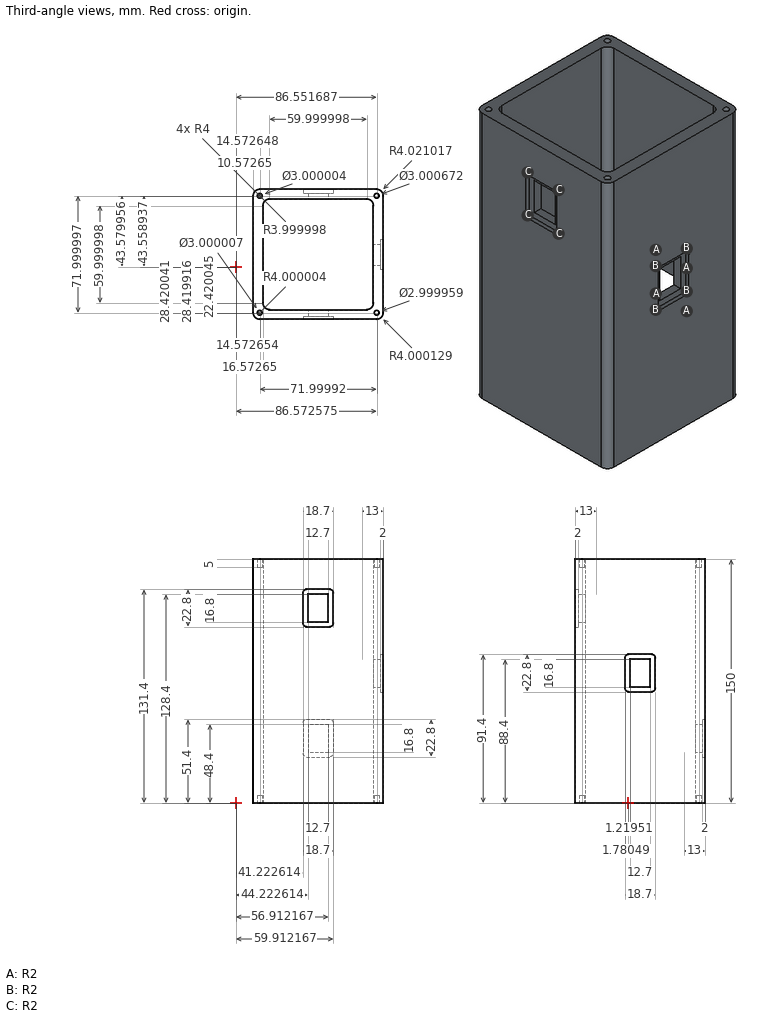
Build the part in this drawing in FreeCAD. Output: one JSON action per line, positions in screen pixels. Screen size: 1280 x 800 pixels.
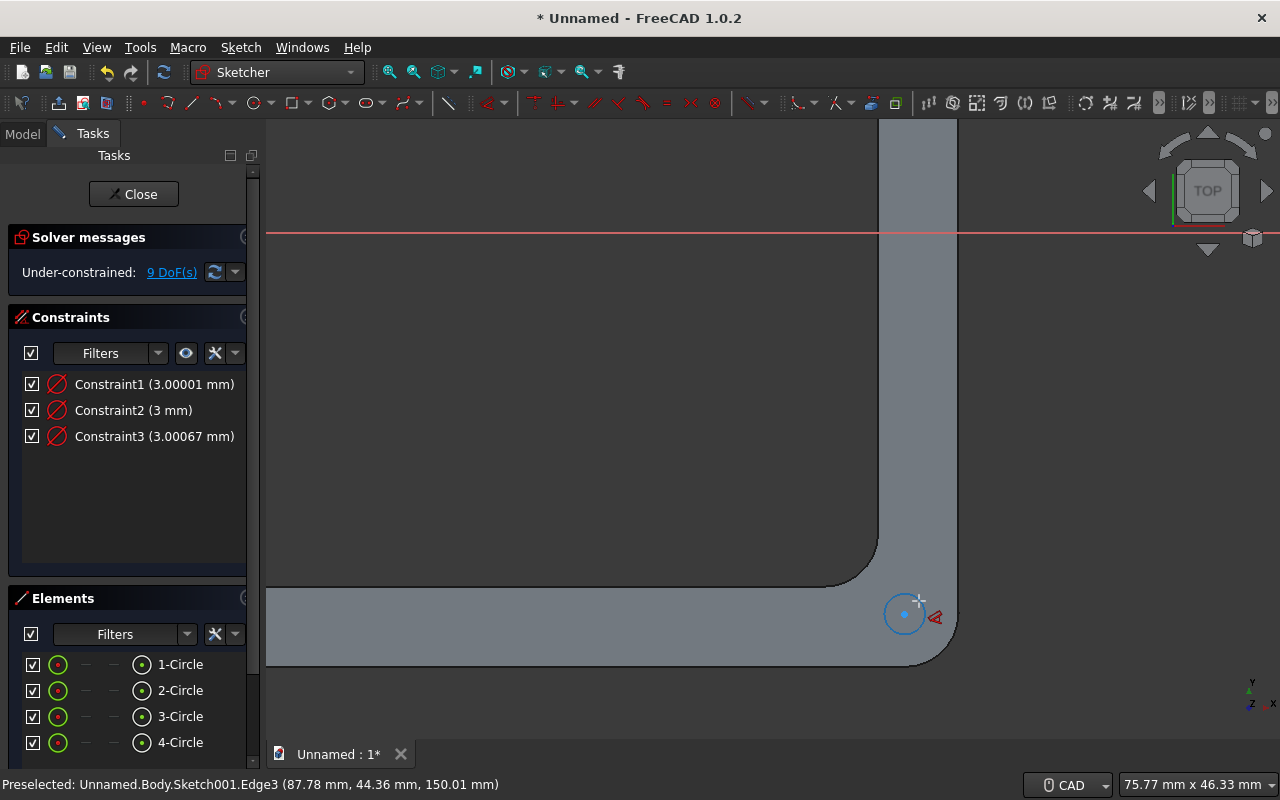
{"action": "left_click", "coordinate": [919, 600]}
{"action": "left_click", "coordinate": [942, 578]}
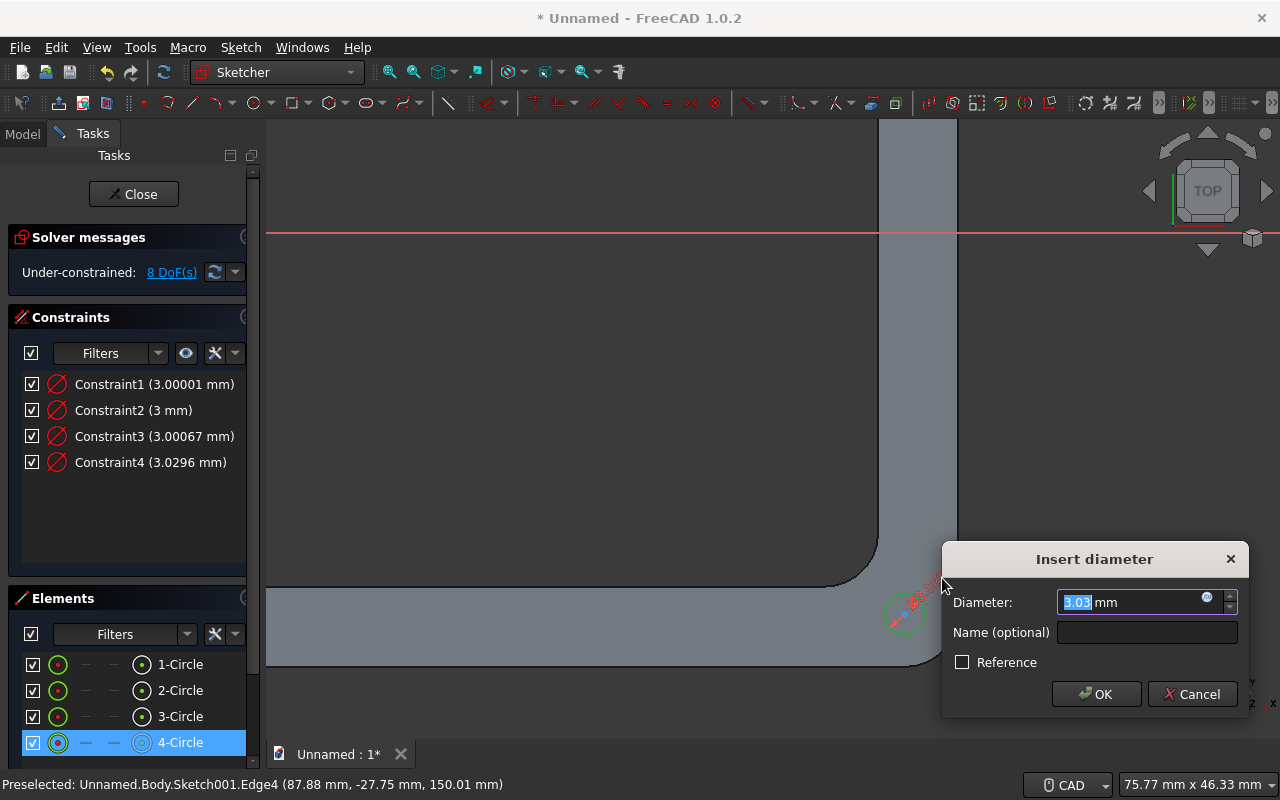
{"action": "type", "text": "2.999959"}
{"action": "key", "text": "Return"}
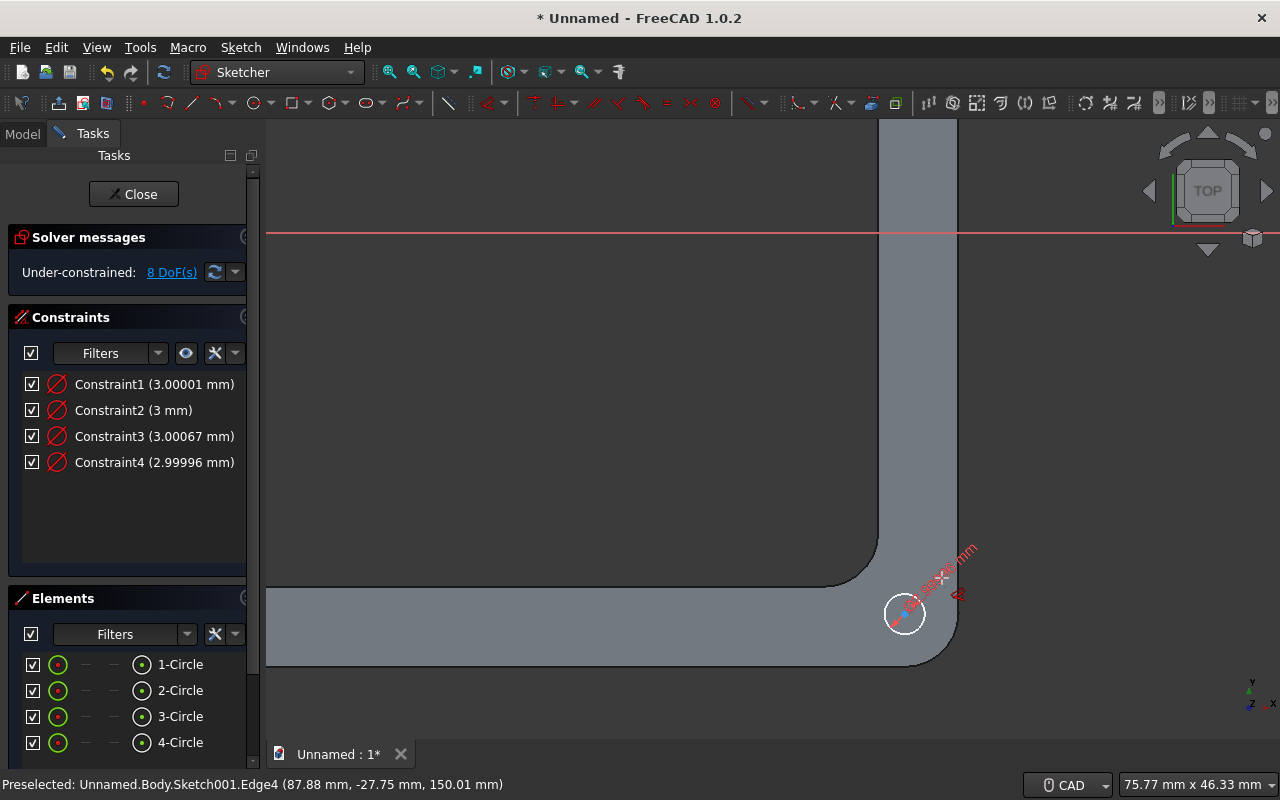
{"action": "scroll", "coordinate": [919, 602], "scroll_direction": "down", "scroll_amount": 5}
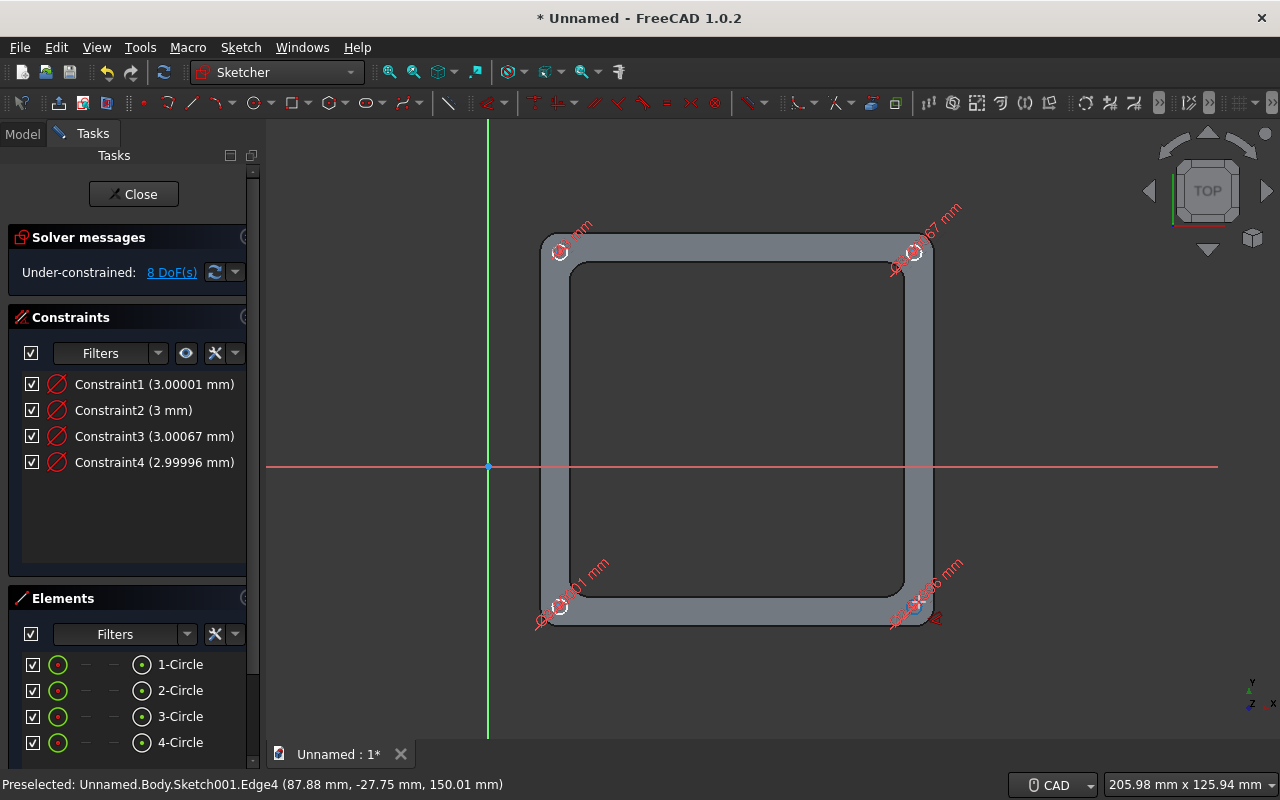
{"action": "left_click", "coordinate": [560, 607]}
{"action": "left_click", "coordinate": [524, 641]}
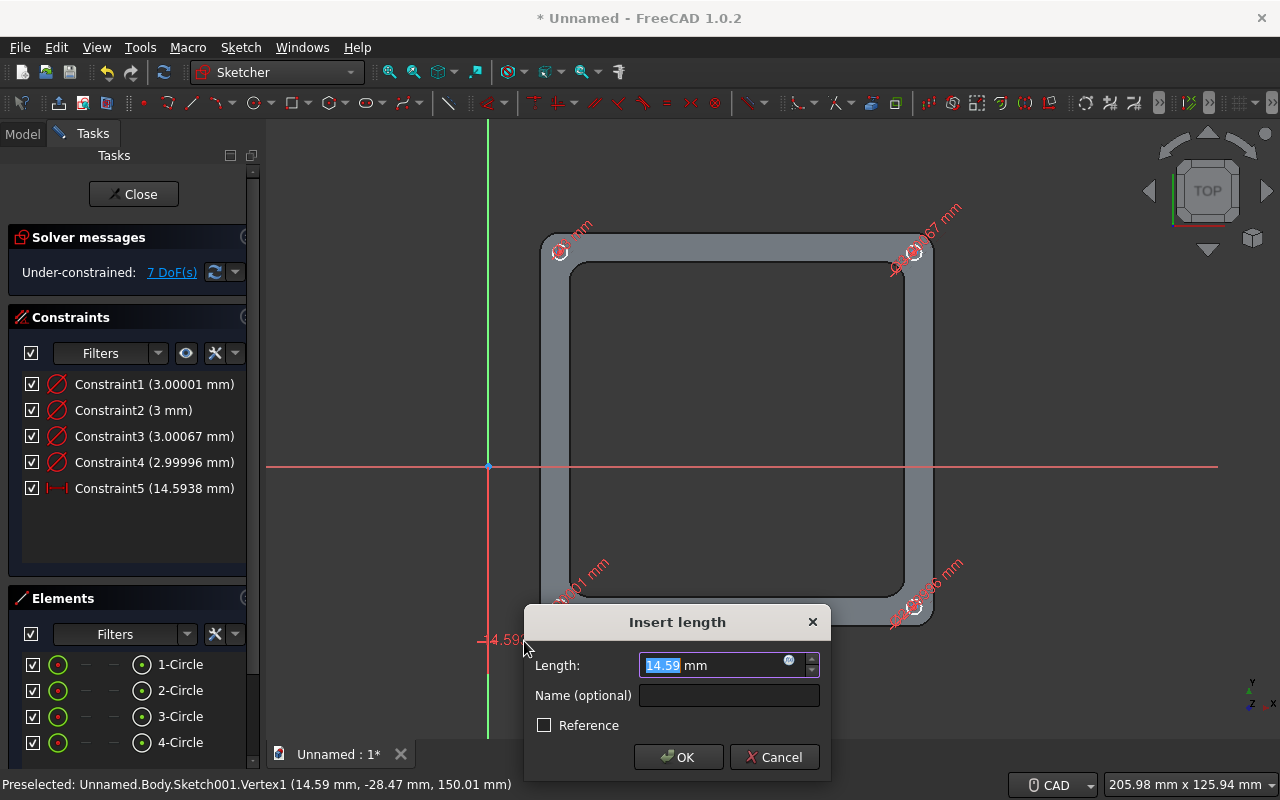
{"action": "type", "text": "14.572654"}
{"action": "key", "text": "Return"}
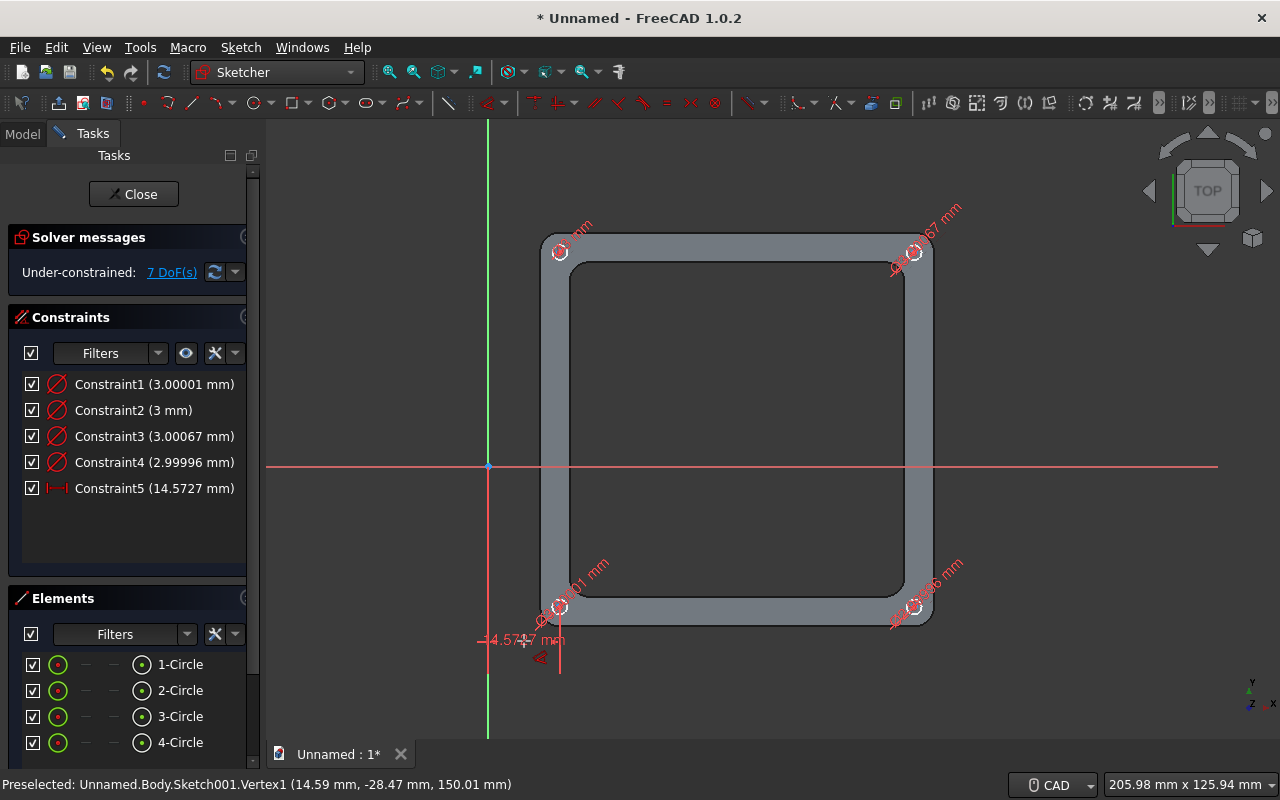
{"action": "left_click", "coordinate": [560, 607]}
{"action": "left_click", "coordinate": [454, 537]}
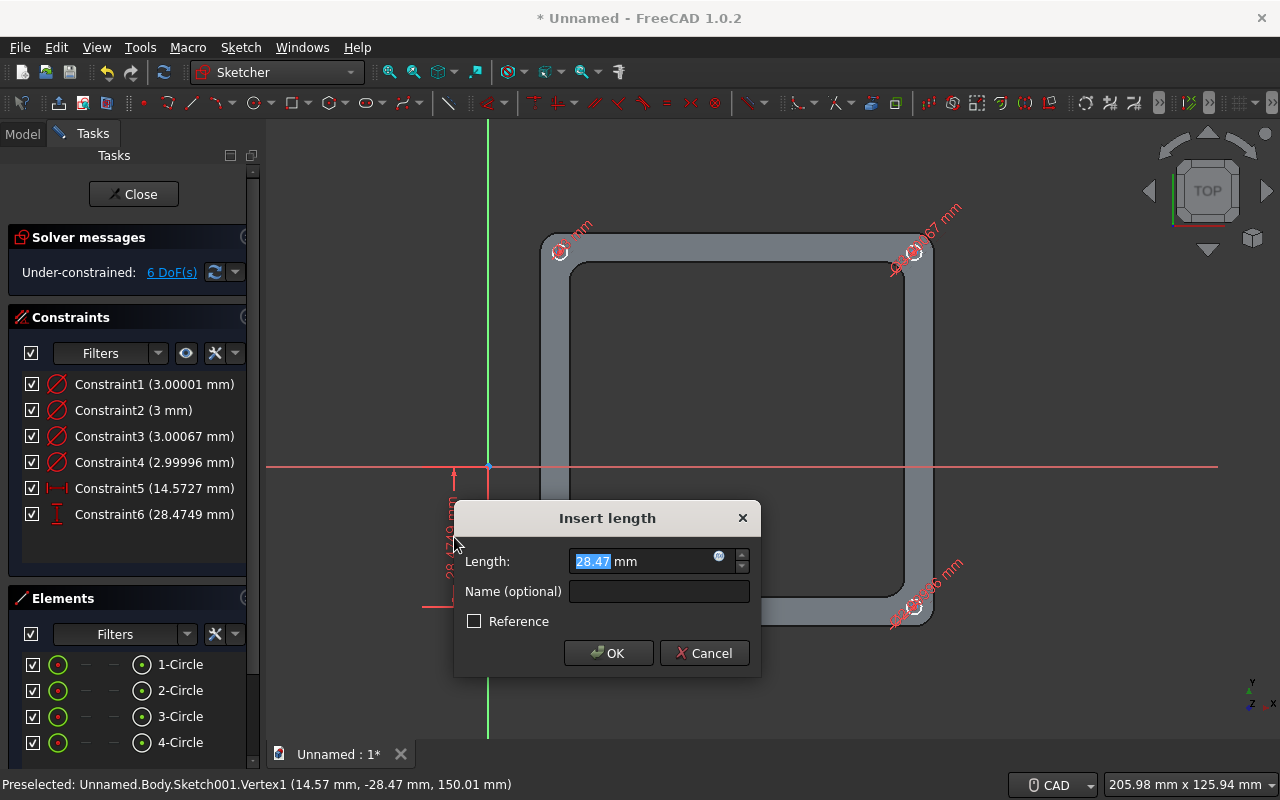
{"action": "type", "text": "28.420041"}
{"action": "key", "text": "Return"}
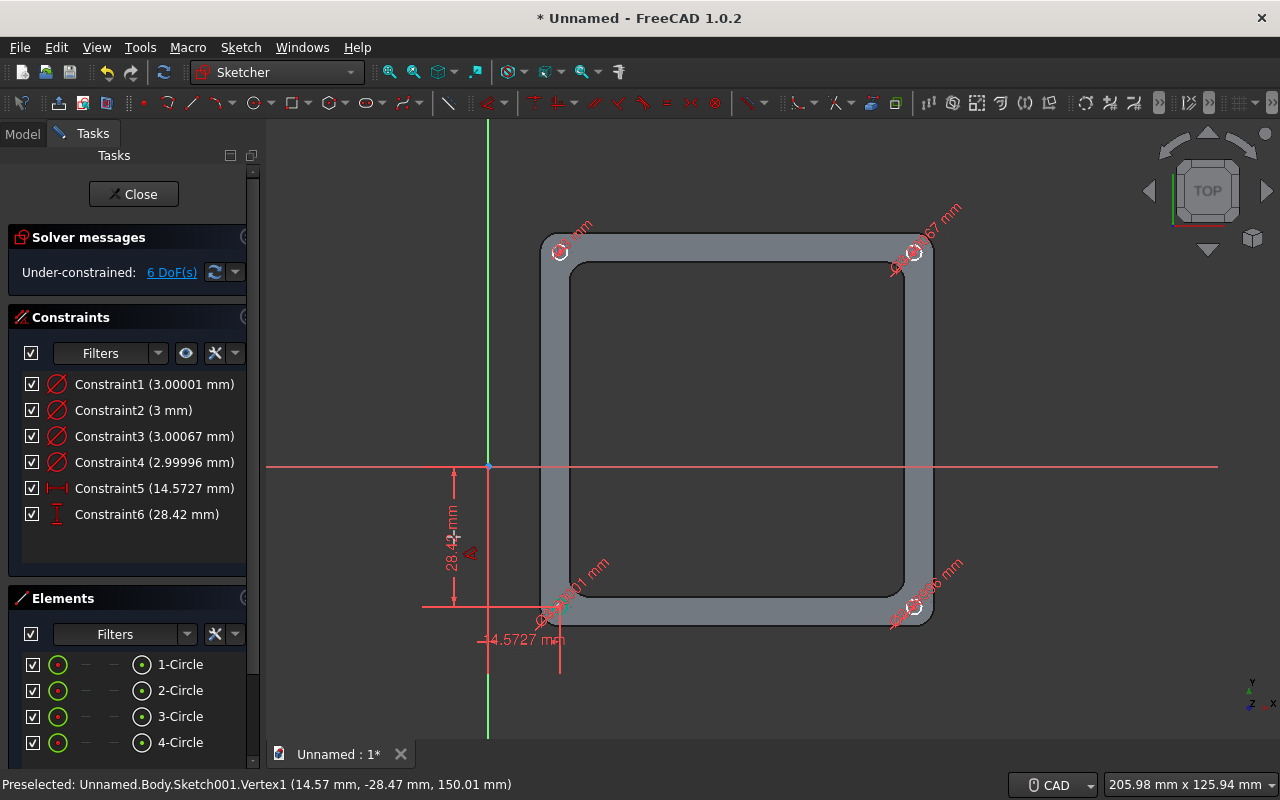
{"action": "left_click", "coordinate": [560, 252]}
{"action": "left_click", "coordinate": [524, 218]}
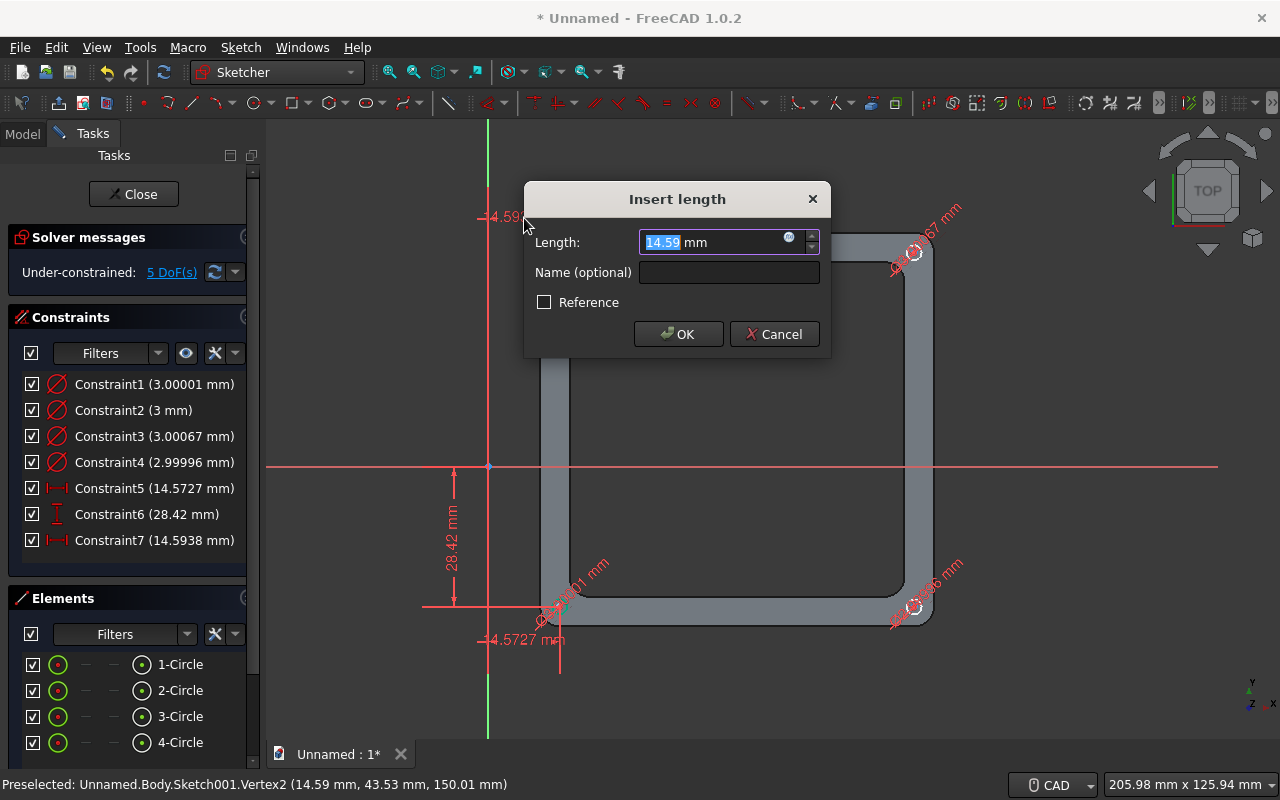
{"action": "type", "text": "14.572648"}
{"action": "key", "text": "Return"}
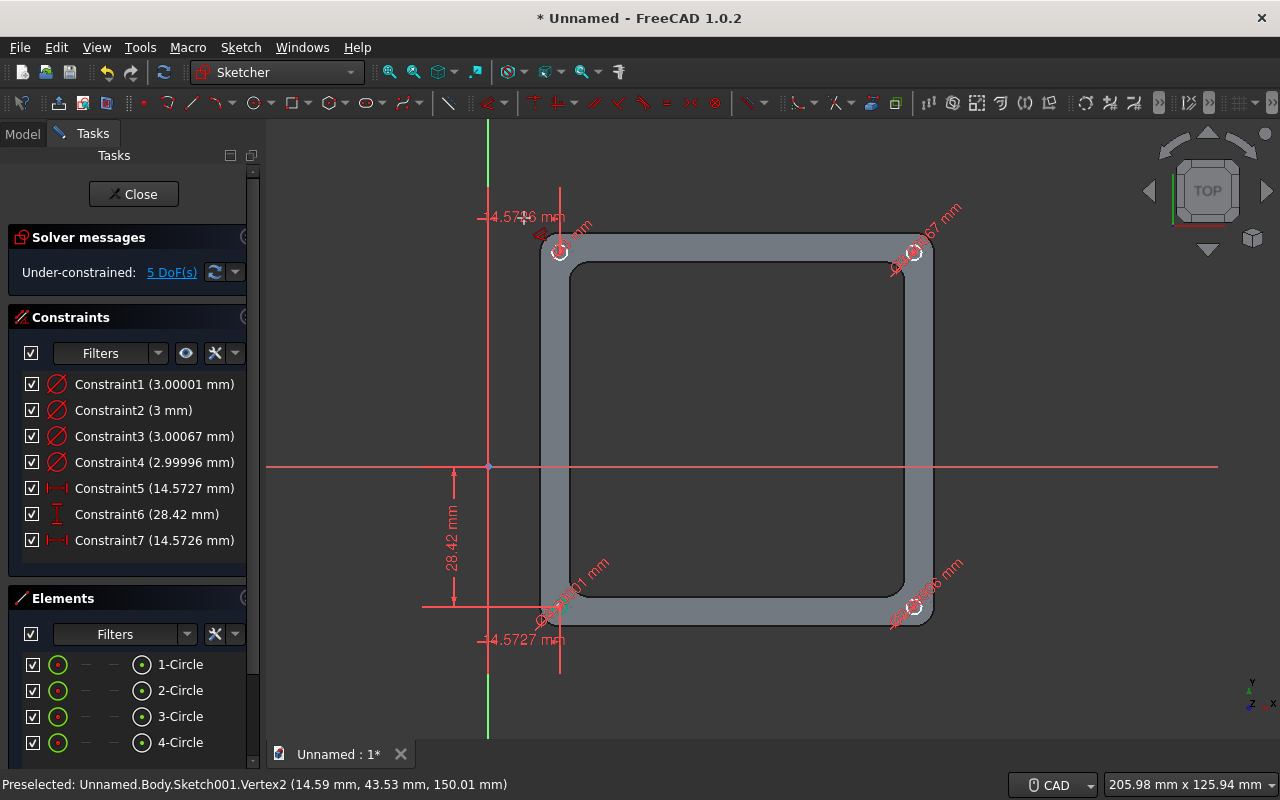
{"action": "left_click", "coordinate": [560, 252]}
{"action": "left_click", "coordinate": [454, 360]}